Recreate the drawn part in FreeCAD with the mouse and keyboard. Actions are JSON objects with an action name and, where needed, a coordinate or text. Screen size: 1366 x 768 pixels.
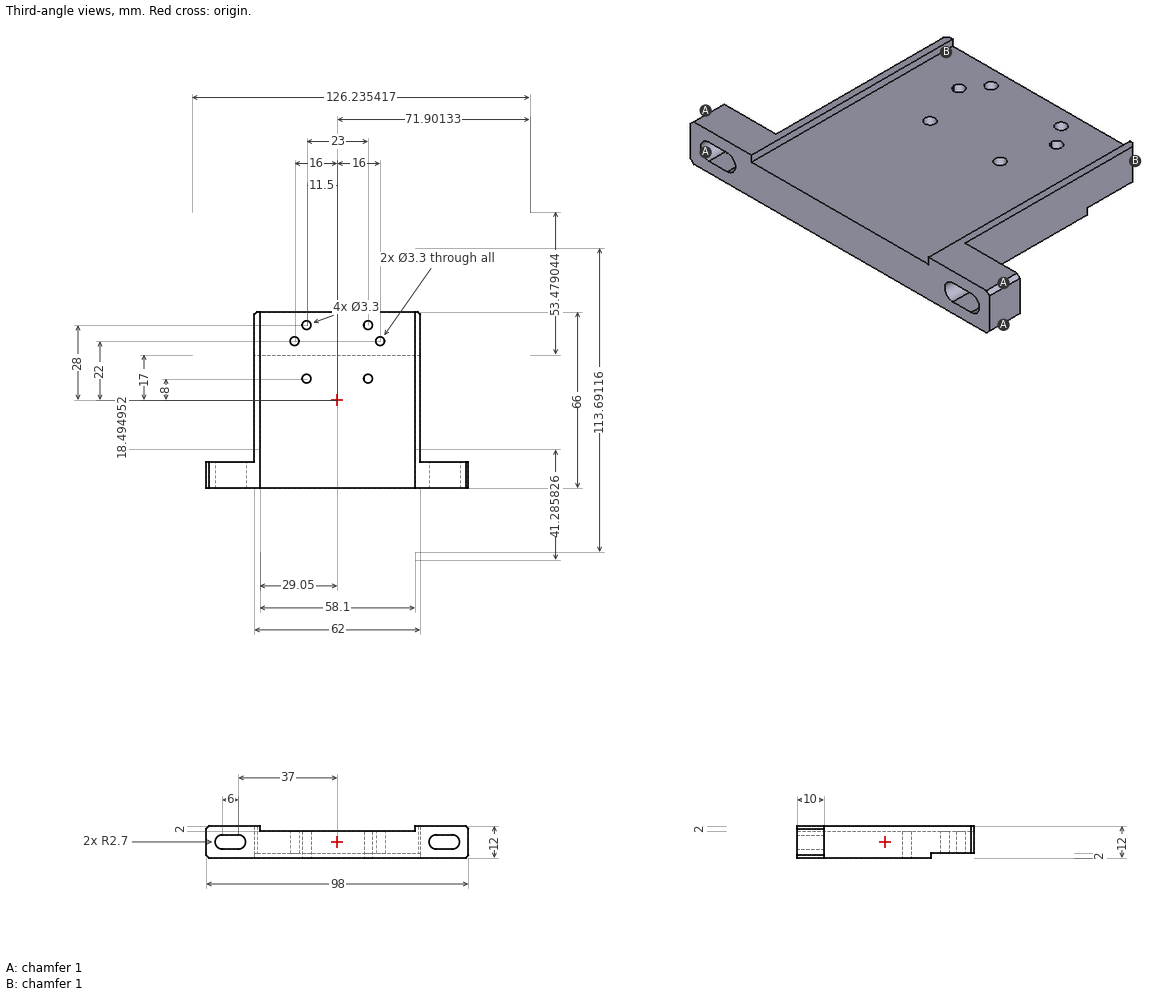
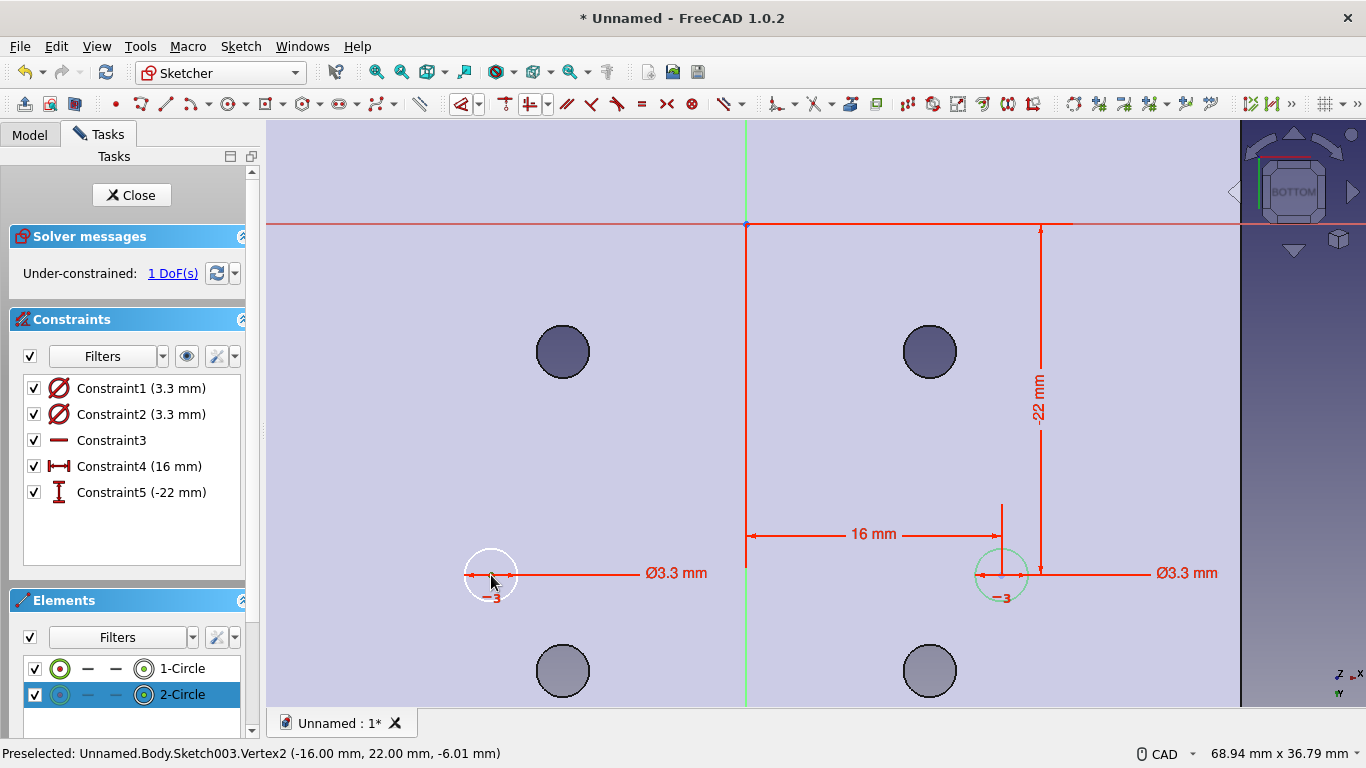
{"action": "left_click", "coordinate": [478, 104]}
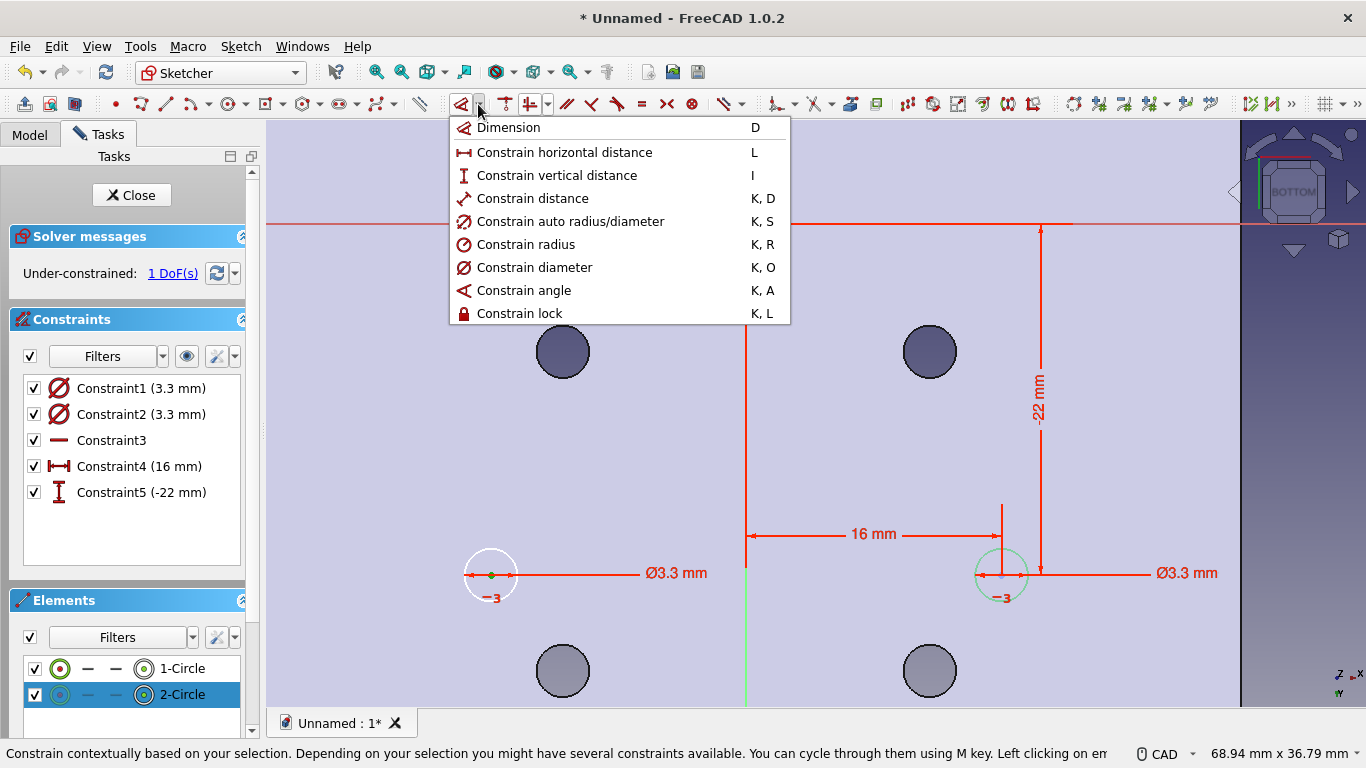
{"action": "left_click", "coordinate": [620, 152]}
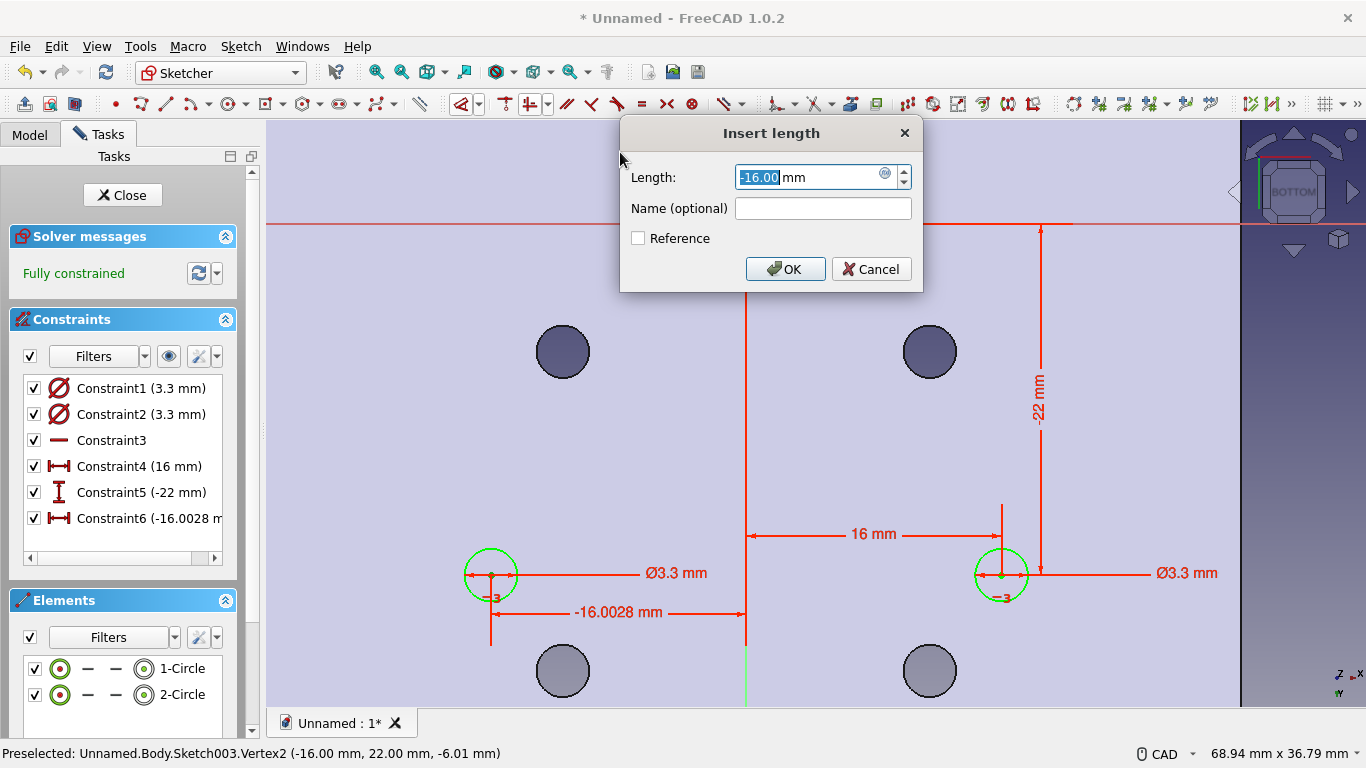
{"action": "type", "text": "-16"}
{"action": "key", "text": "Return"}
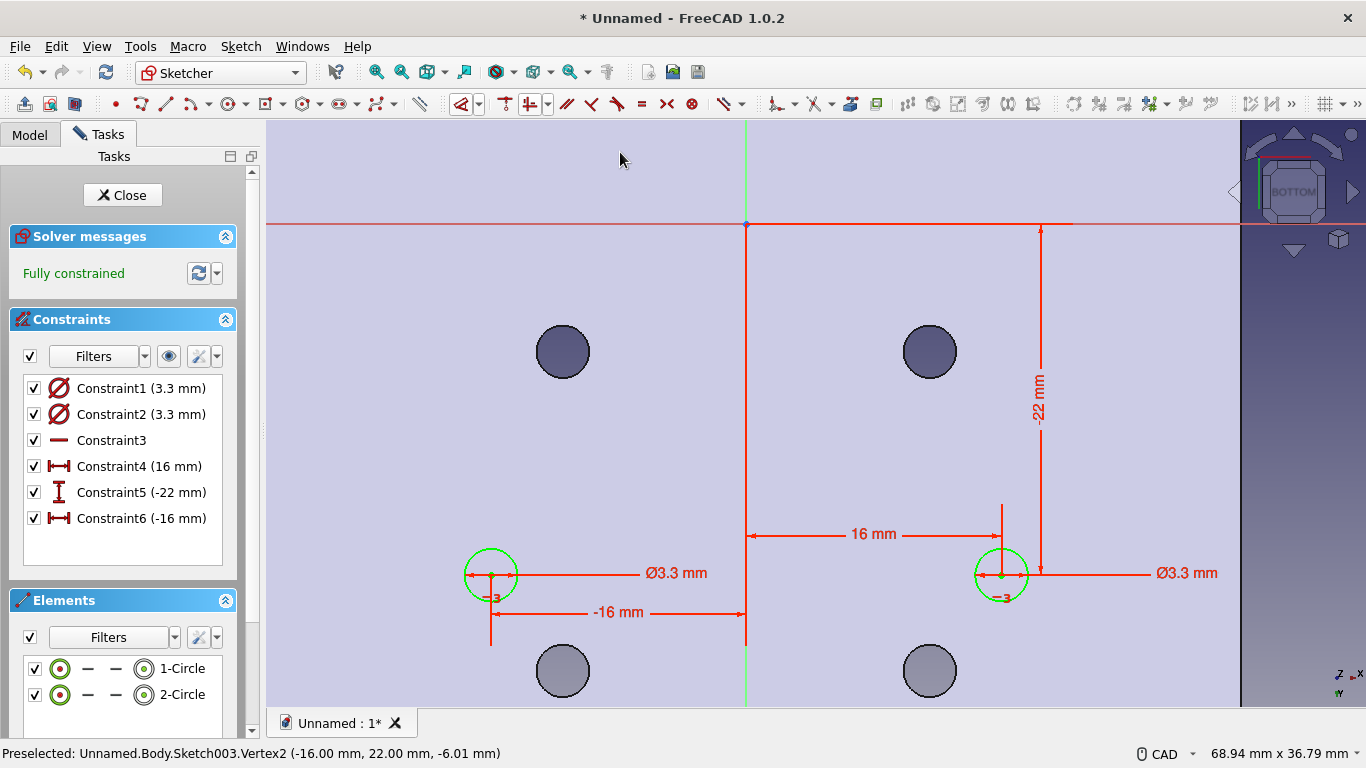
{"action": "left_click", "coordinate": [123, 195]}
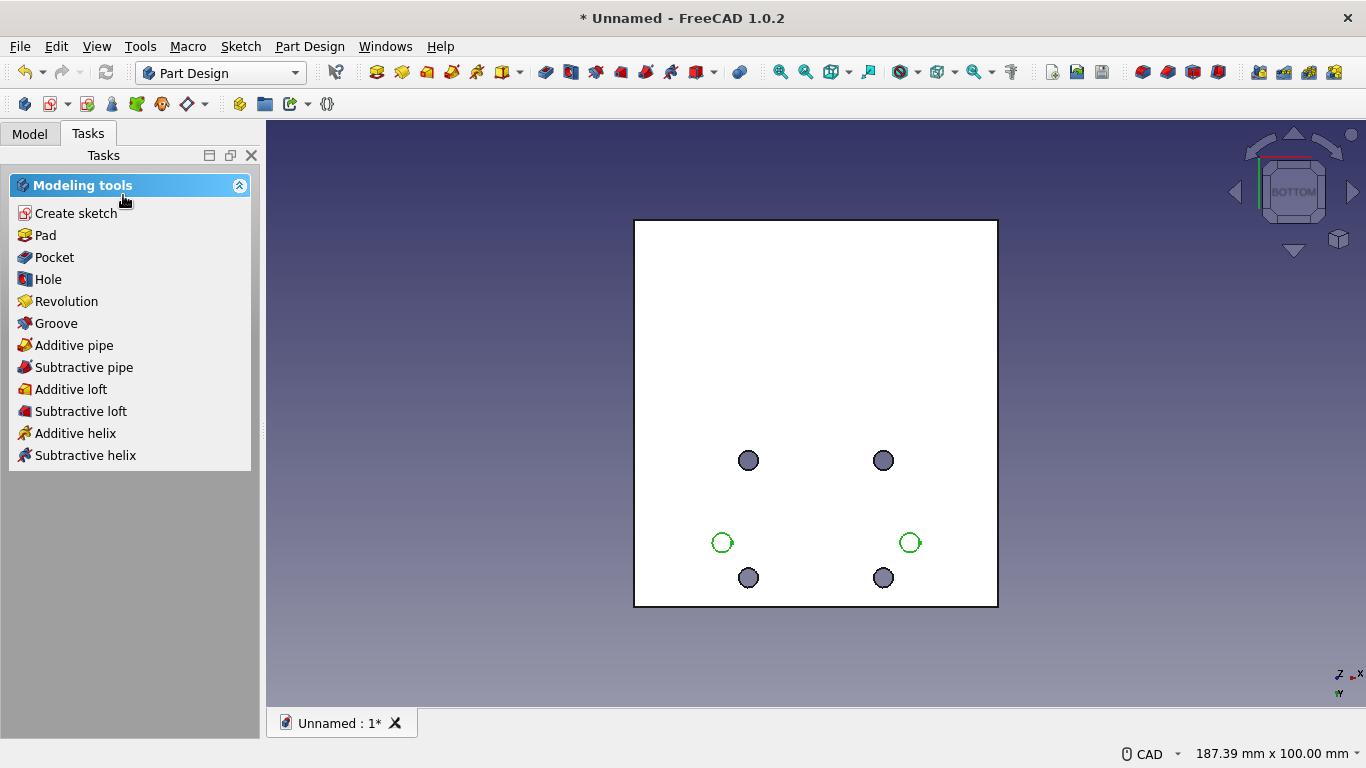
{"action": "left_click", "coordinate": [571, 72]}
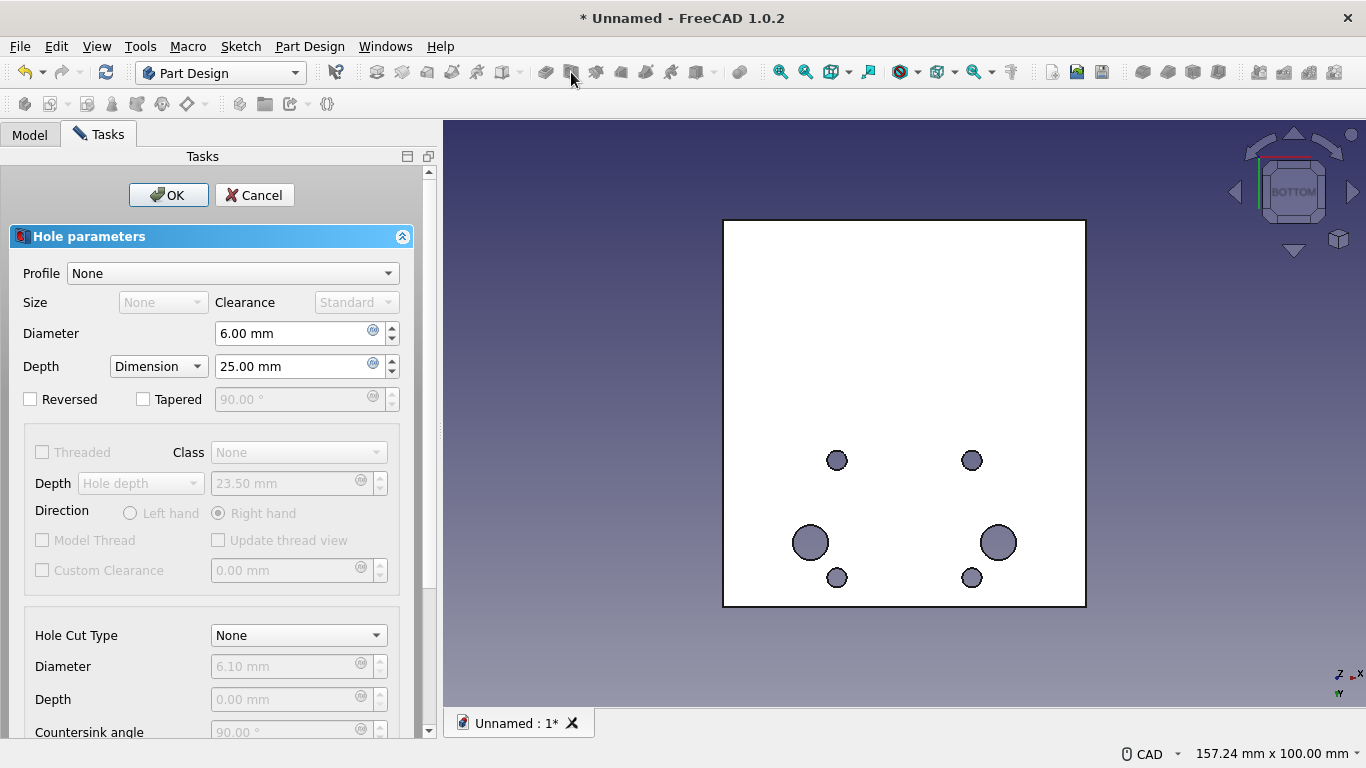
{"action": "triple_click", "coordinate": [300, 334]}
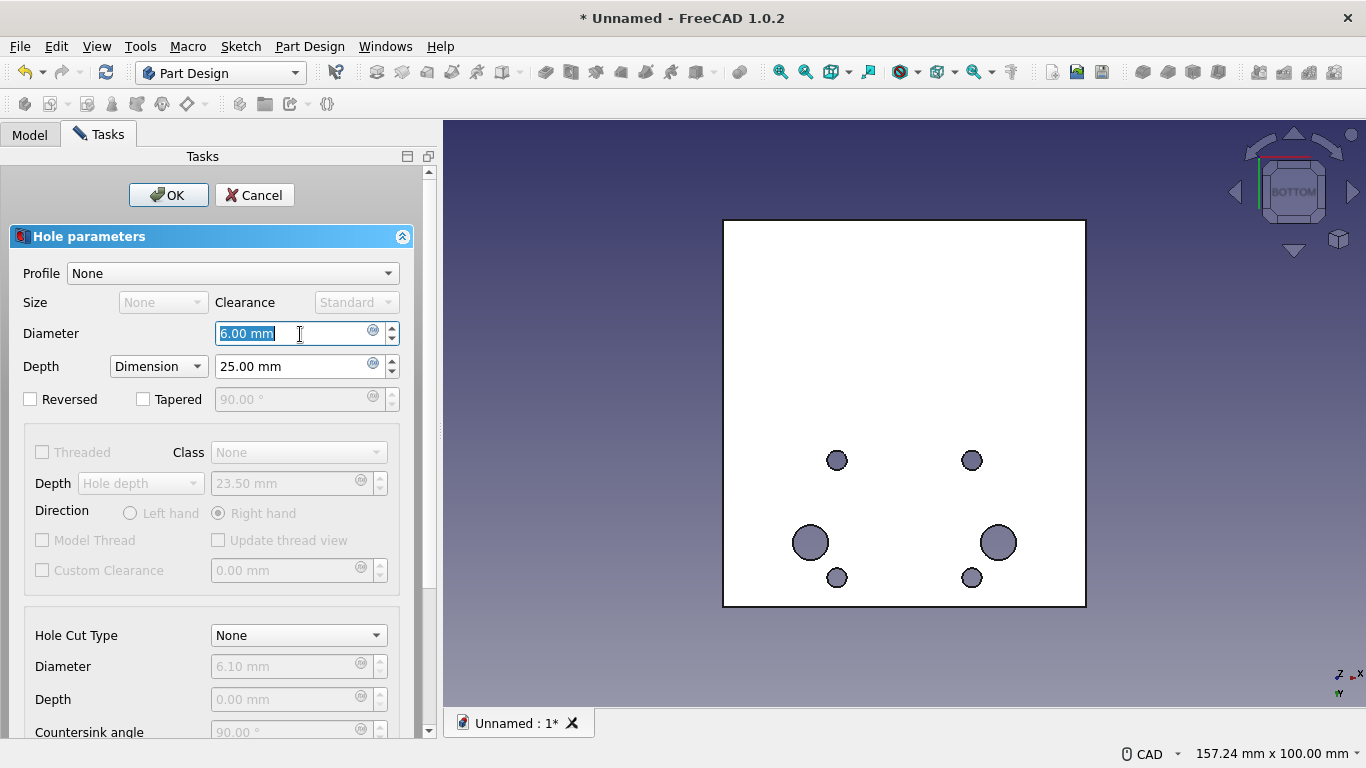
{"action": "type", "text": "3.3"}
{"action": "key", "text": "Tab"}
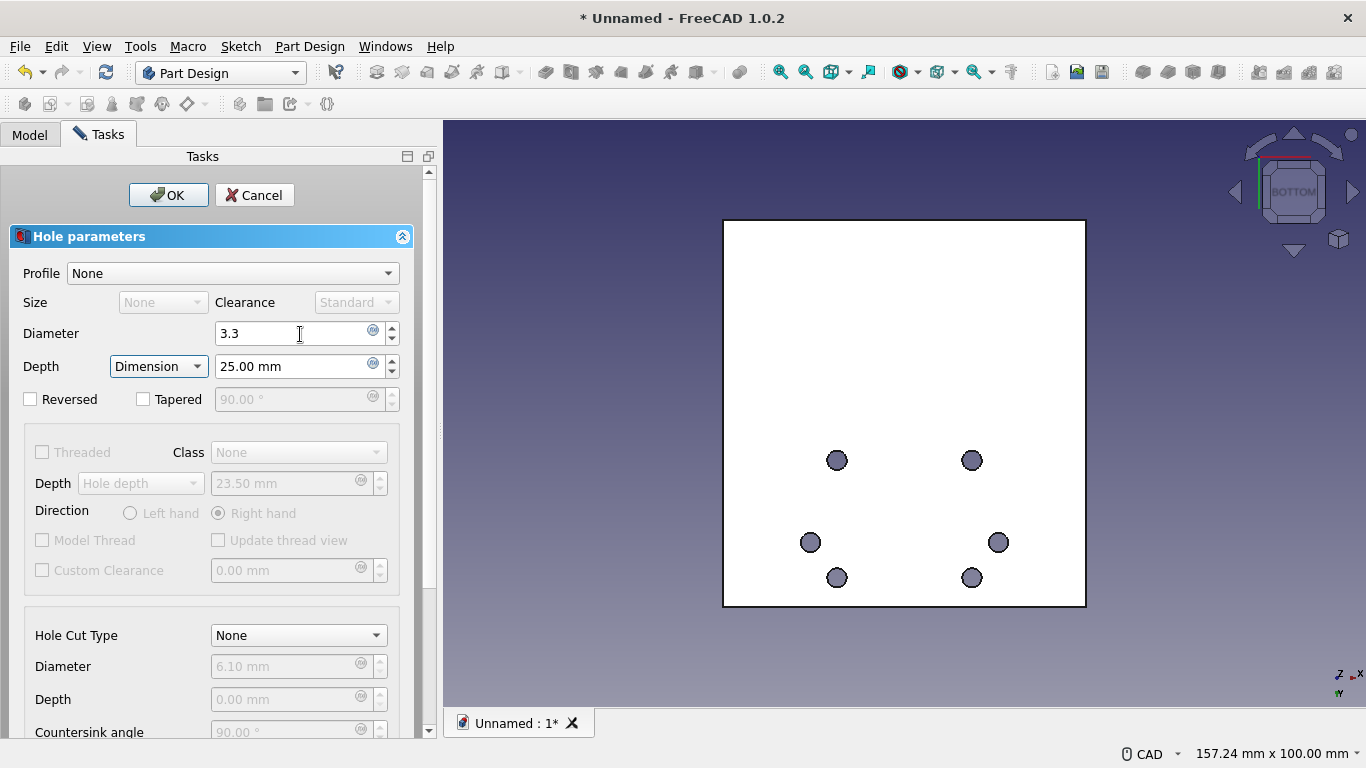
{"action": "left_click", "coordinate": [160, 366]}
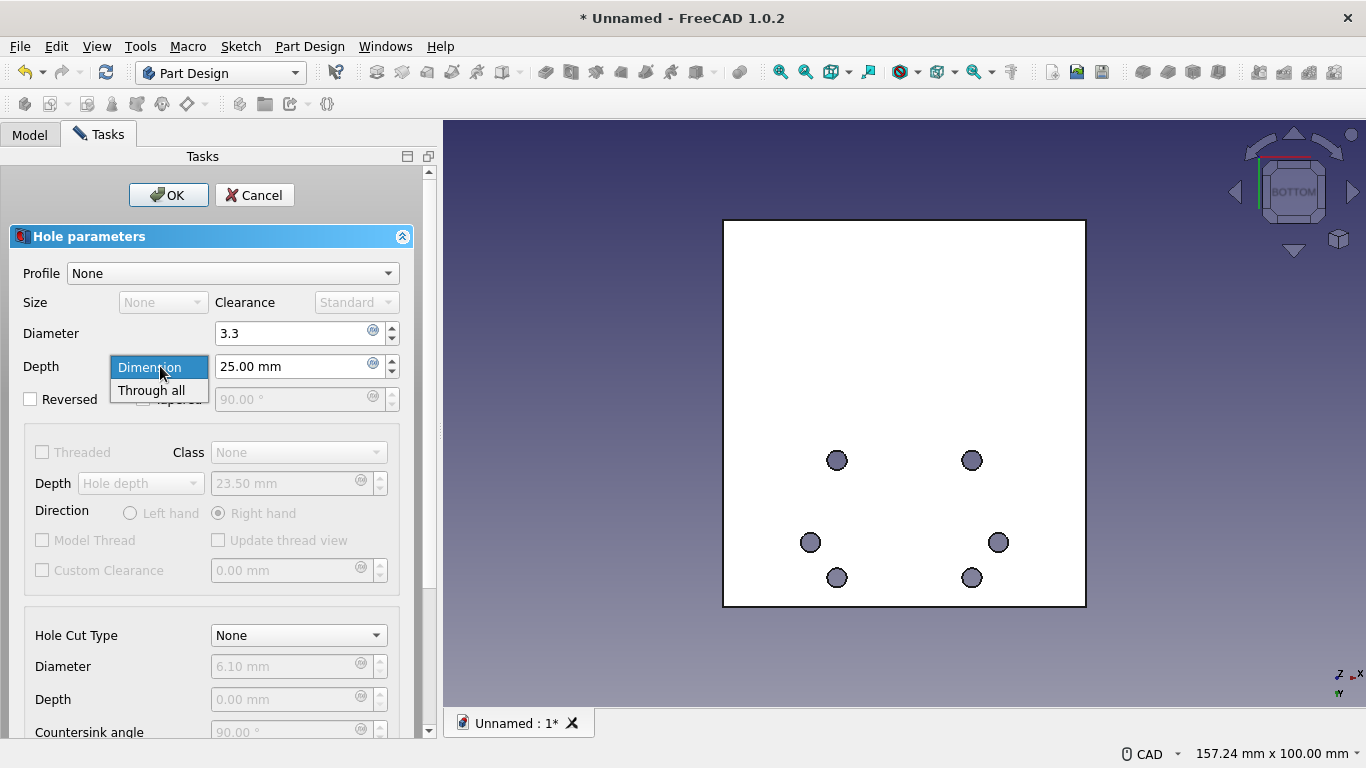
{"action": "left_click", "coordinate": [158, 390]}